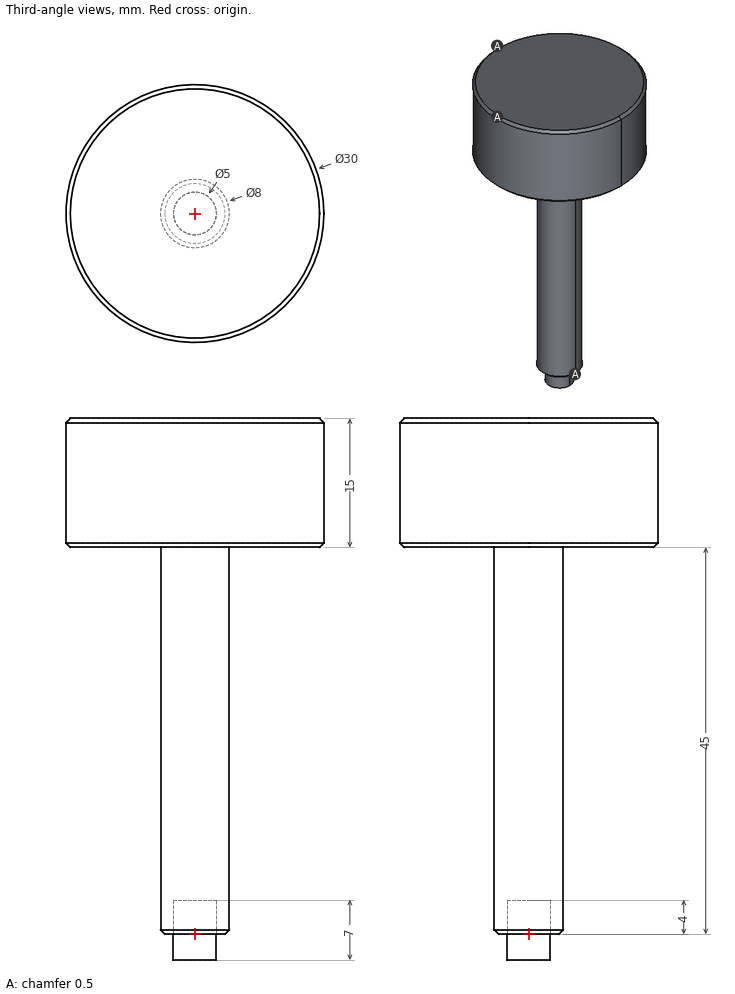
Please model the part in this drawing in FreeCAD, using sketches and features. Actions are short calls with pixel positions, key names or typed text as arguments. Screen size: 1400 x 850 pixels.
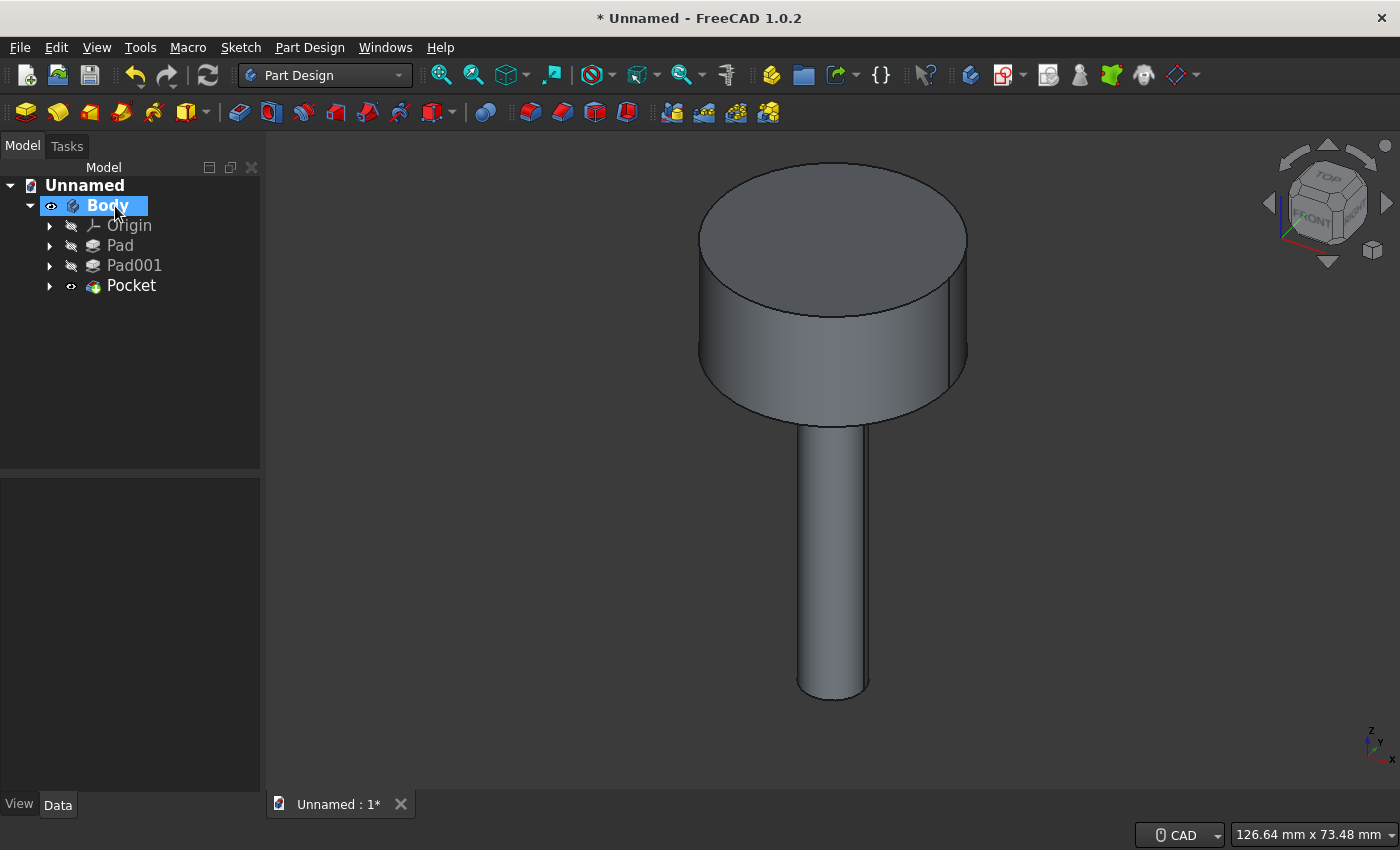
click(733, 401)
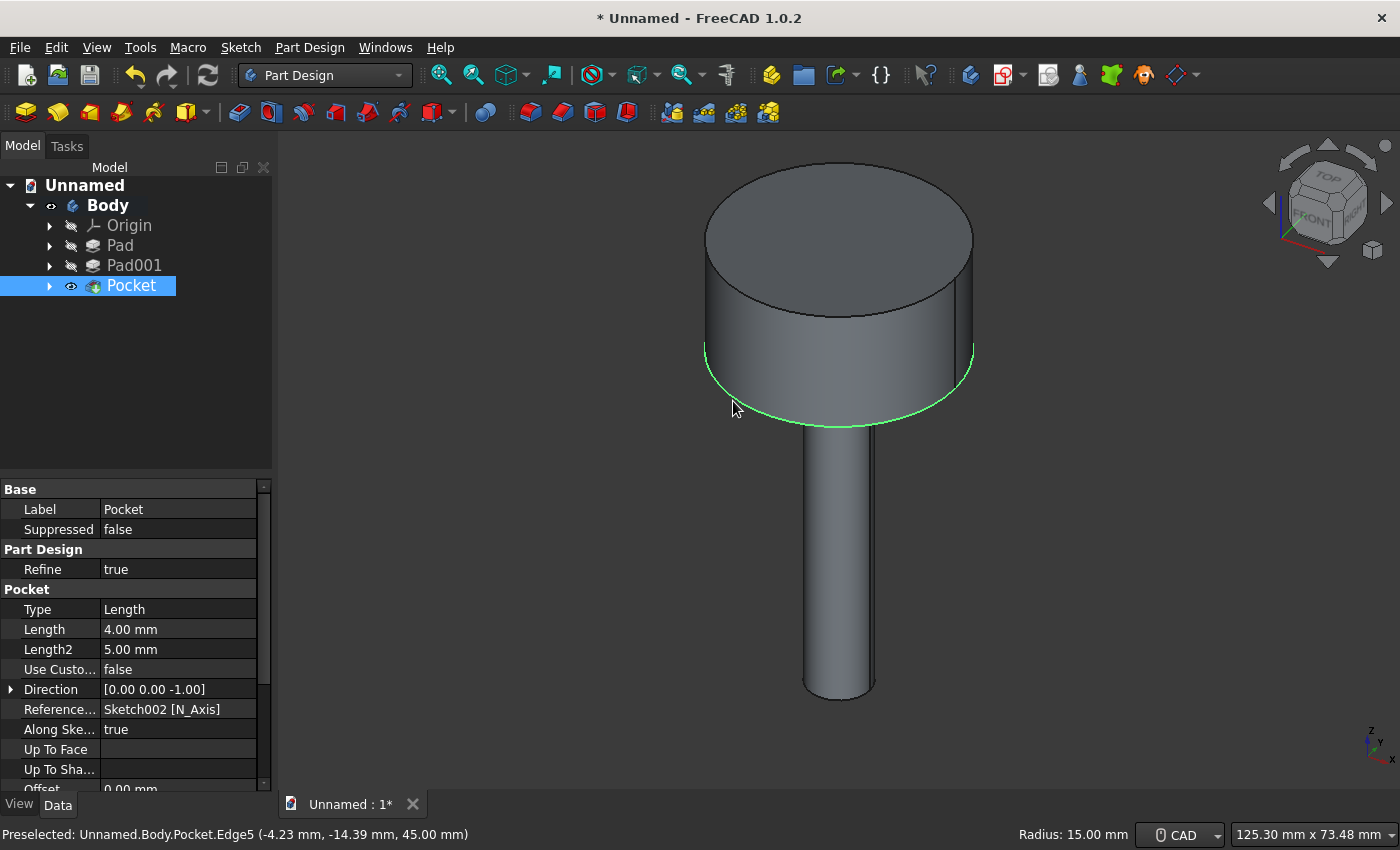
click(705, 247, ctrl)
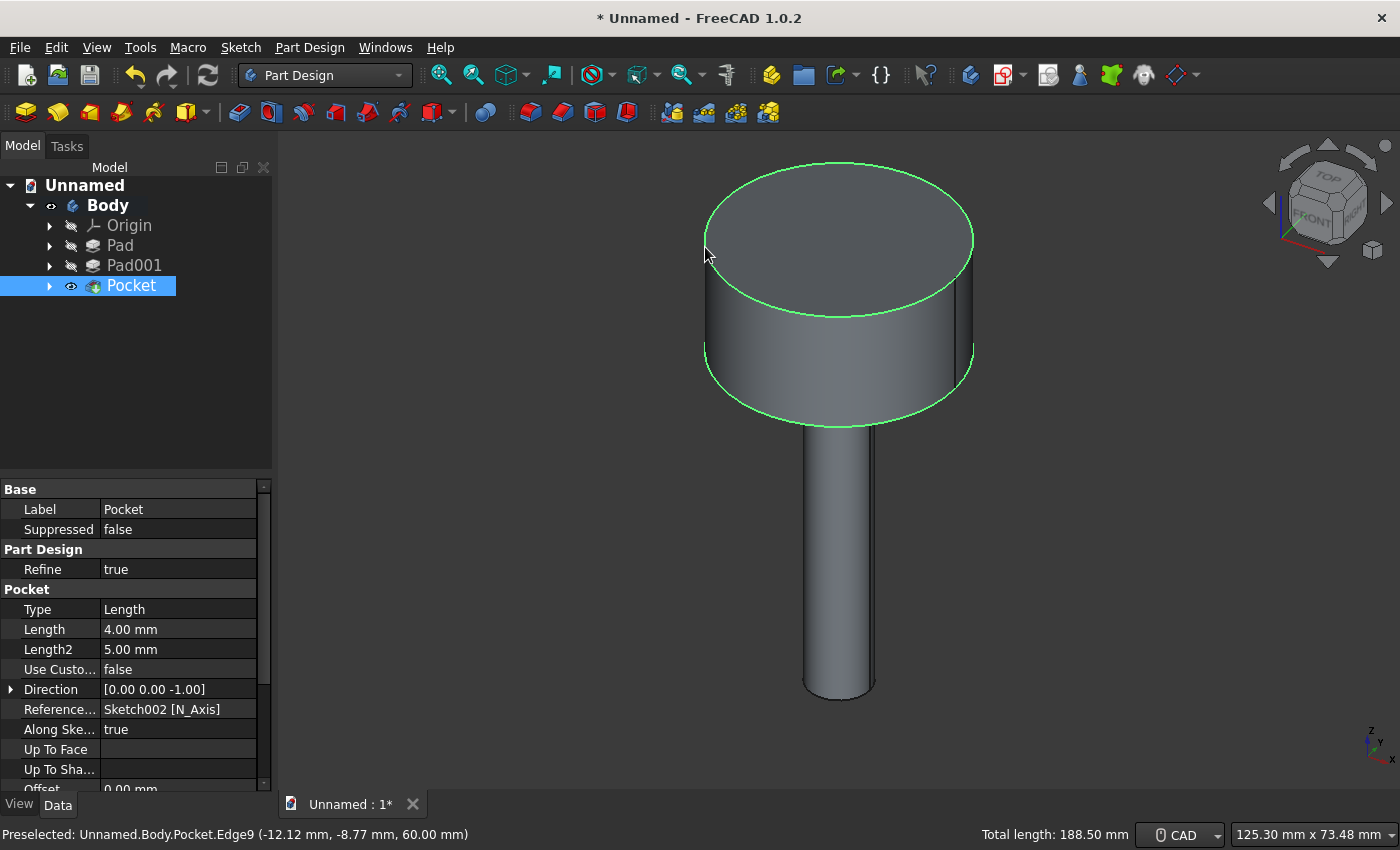
key(0)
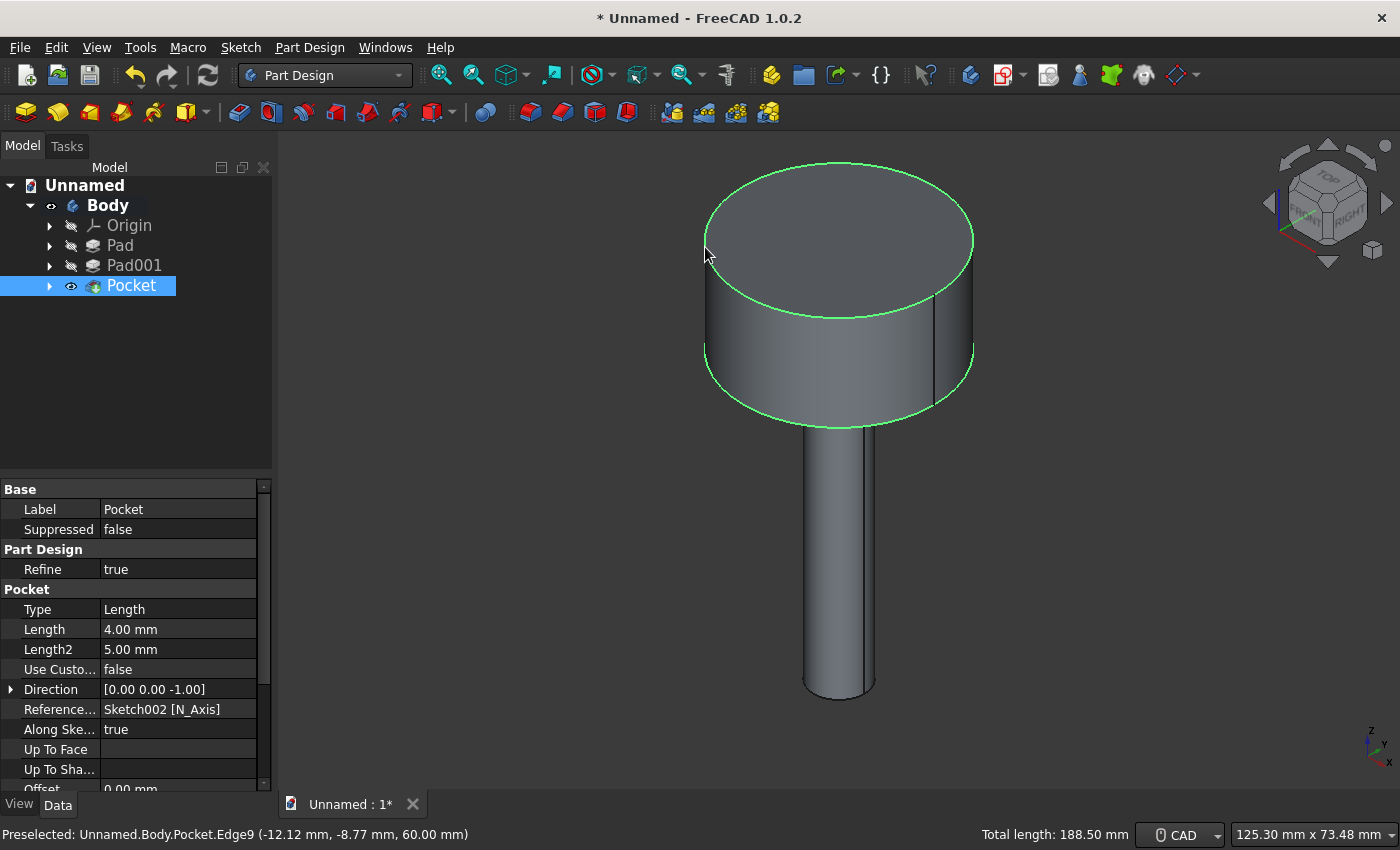
click(442, 76)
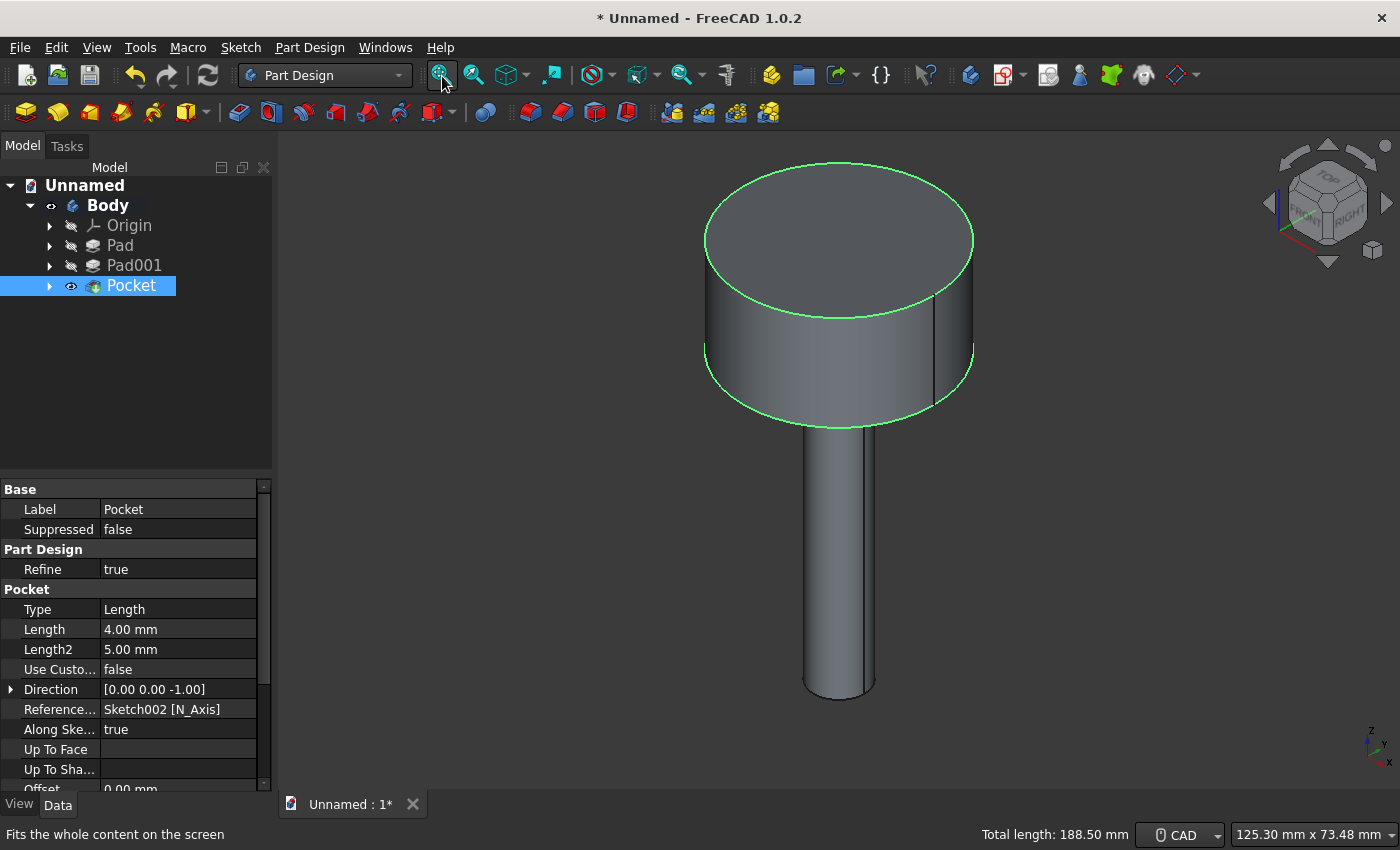
key(2)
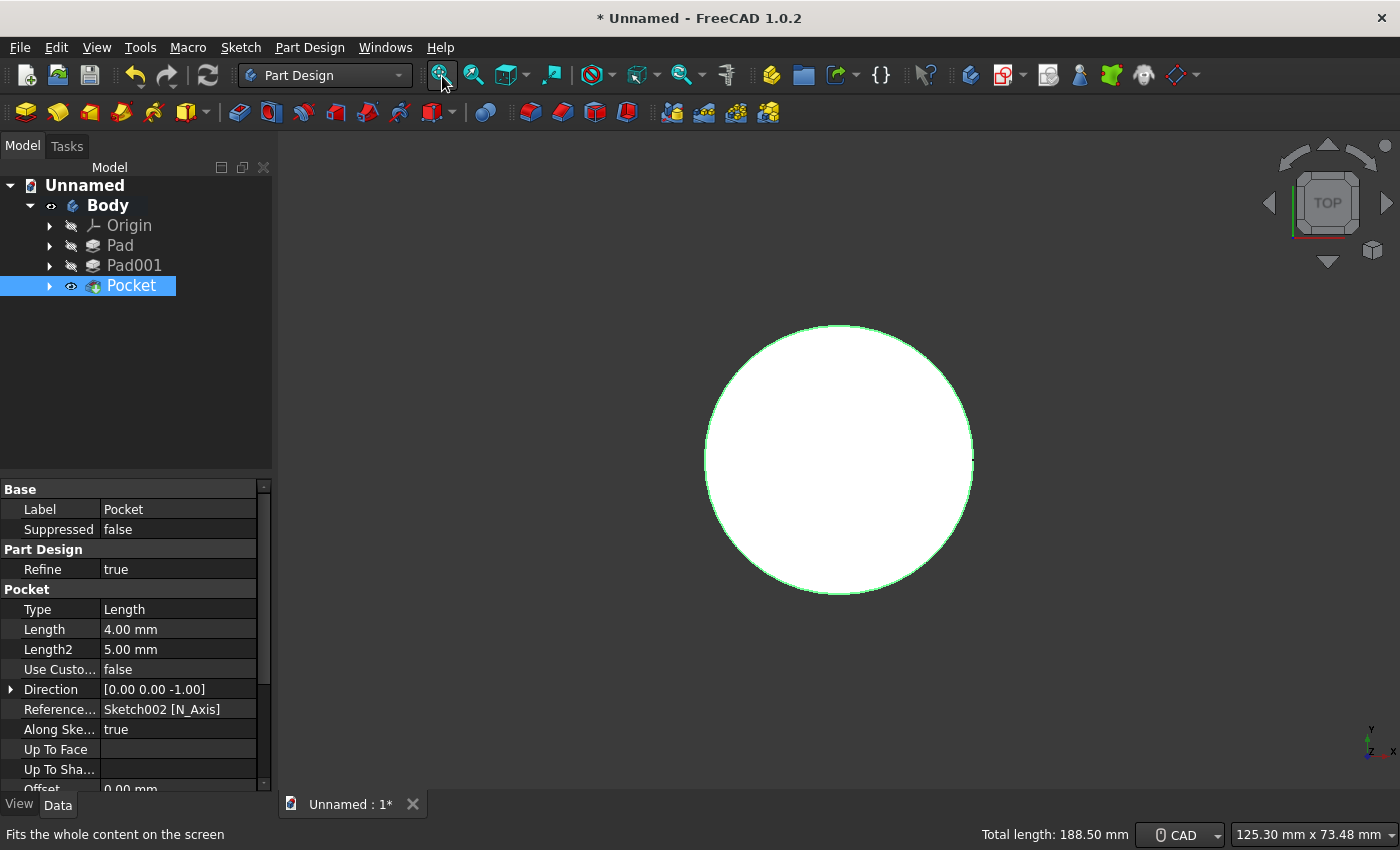
key(v)
key(f)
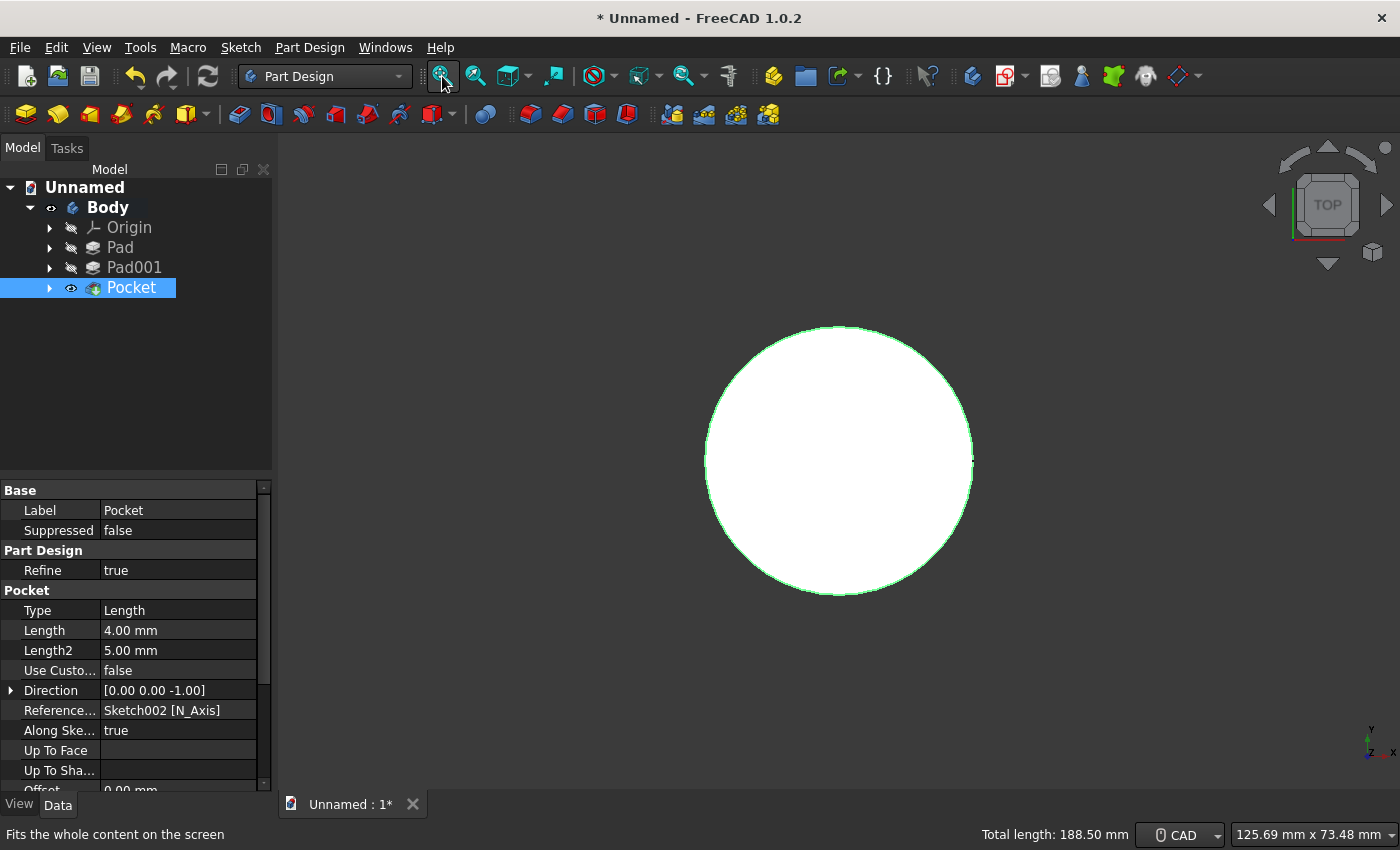
key(1)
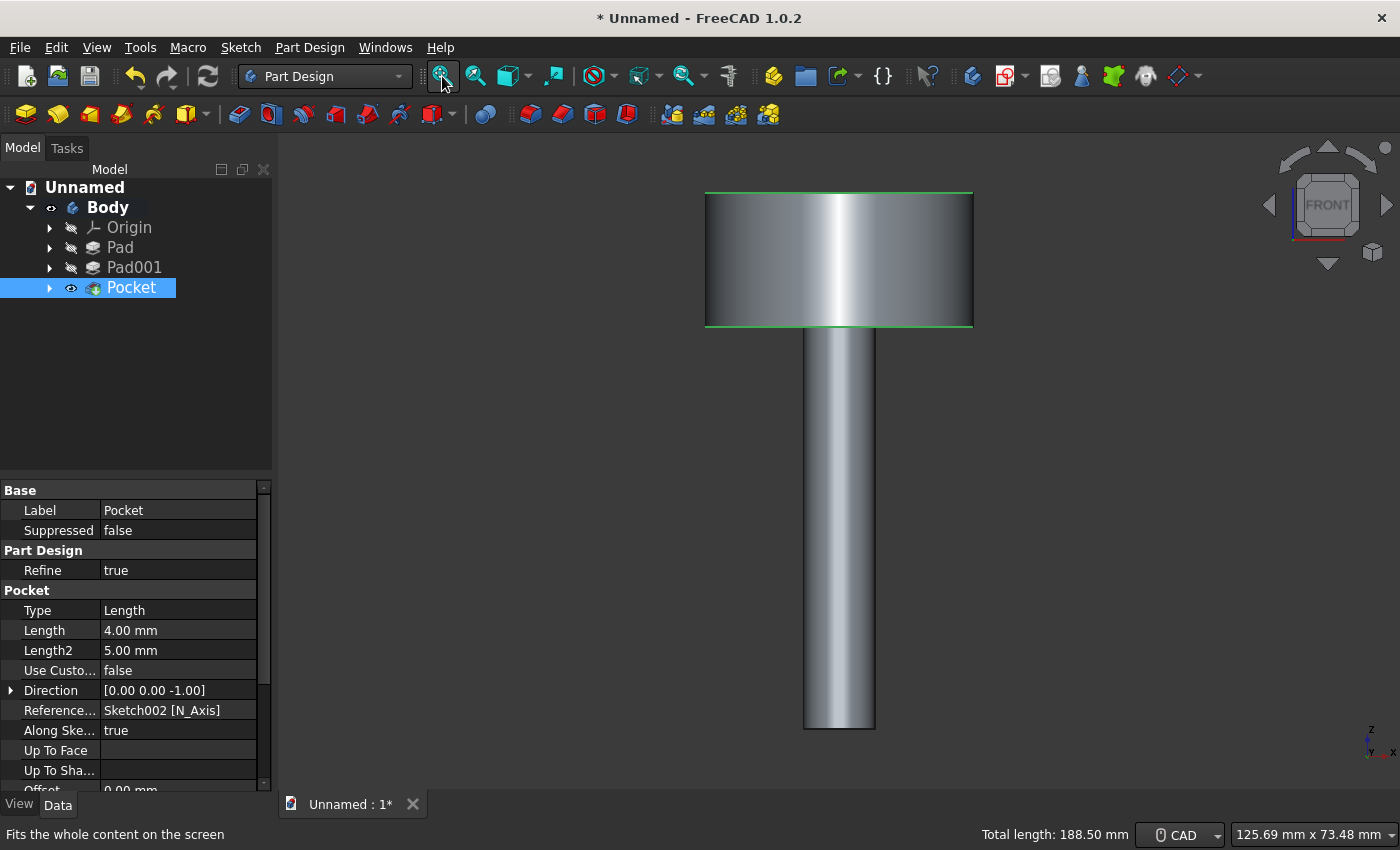
click(810, 728, ctrl)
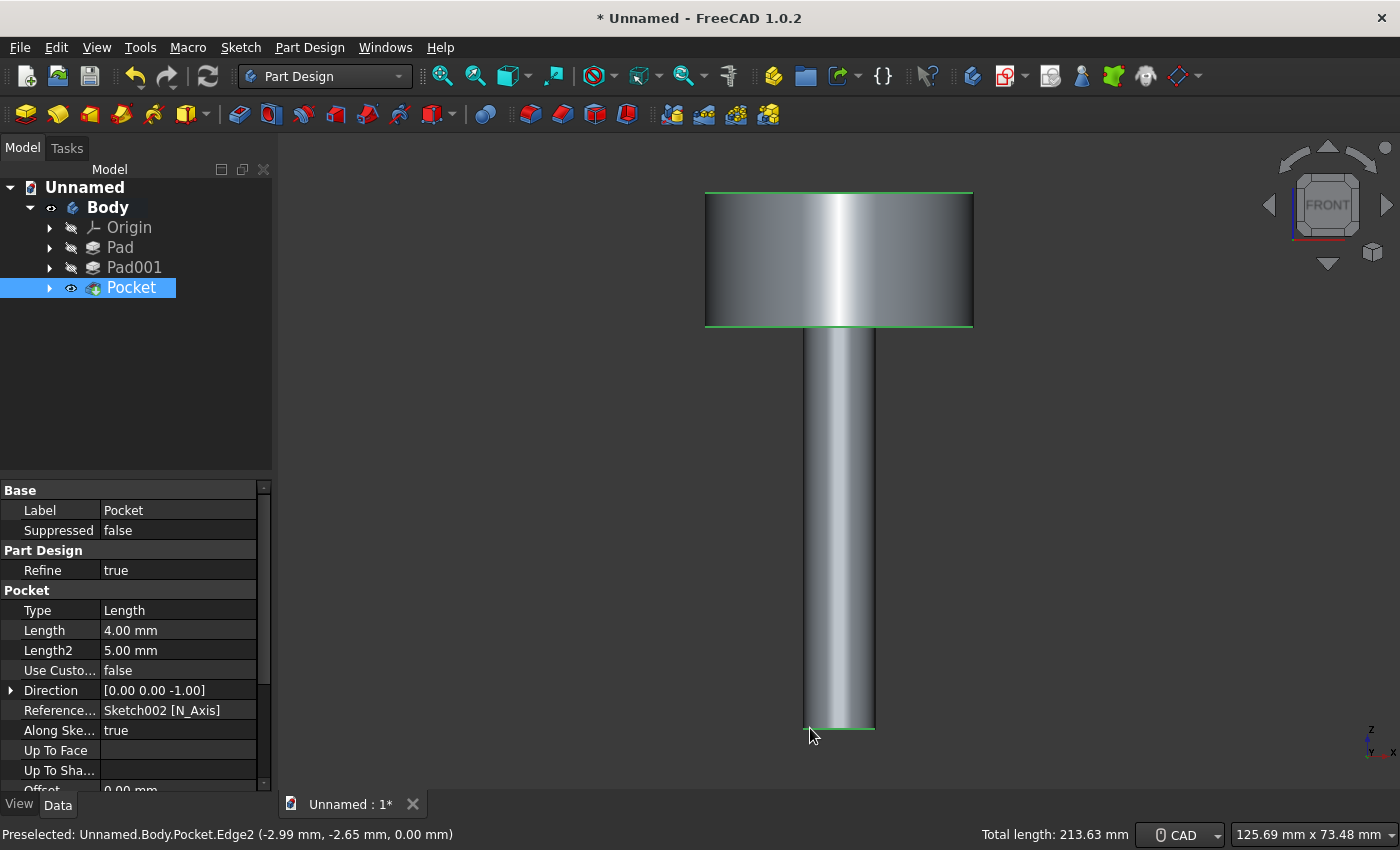
click(564, 114)